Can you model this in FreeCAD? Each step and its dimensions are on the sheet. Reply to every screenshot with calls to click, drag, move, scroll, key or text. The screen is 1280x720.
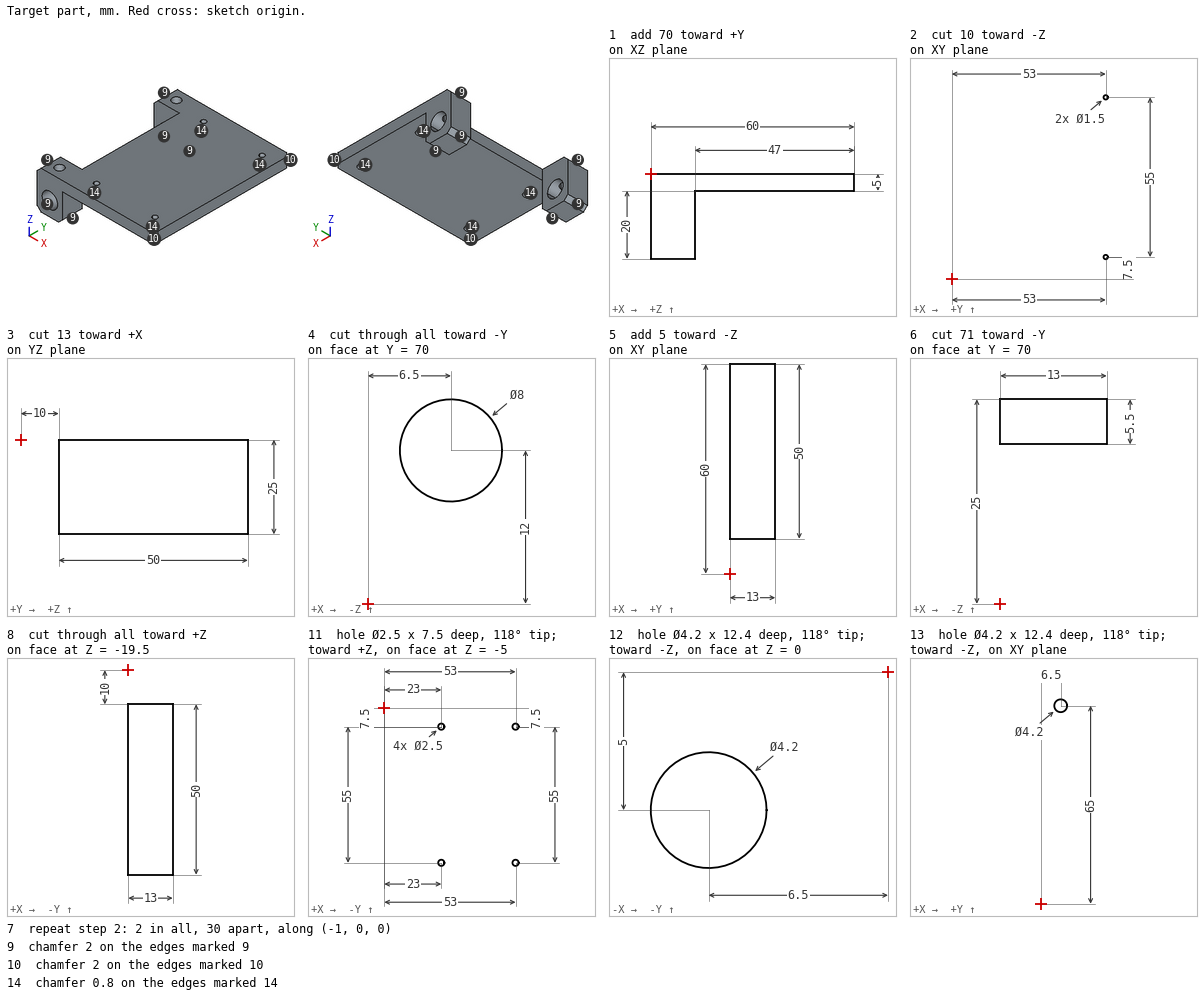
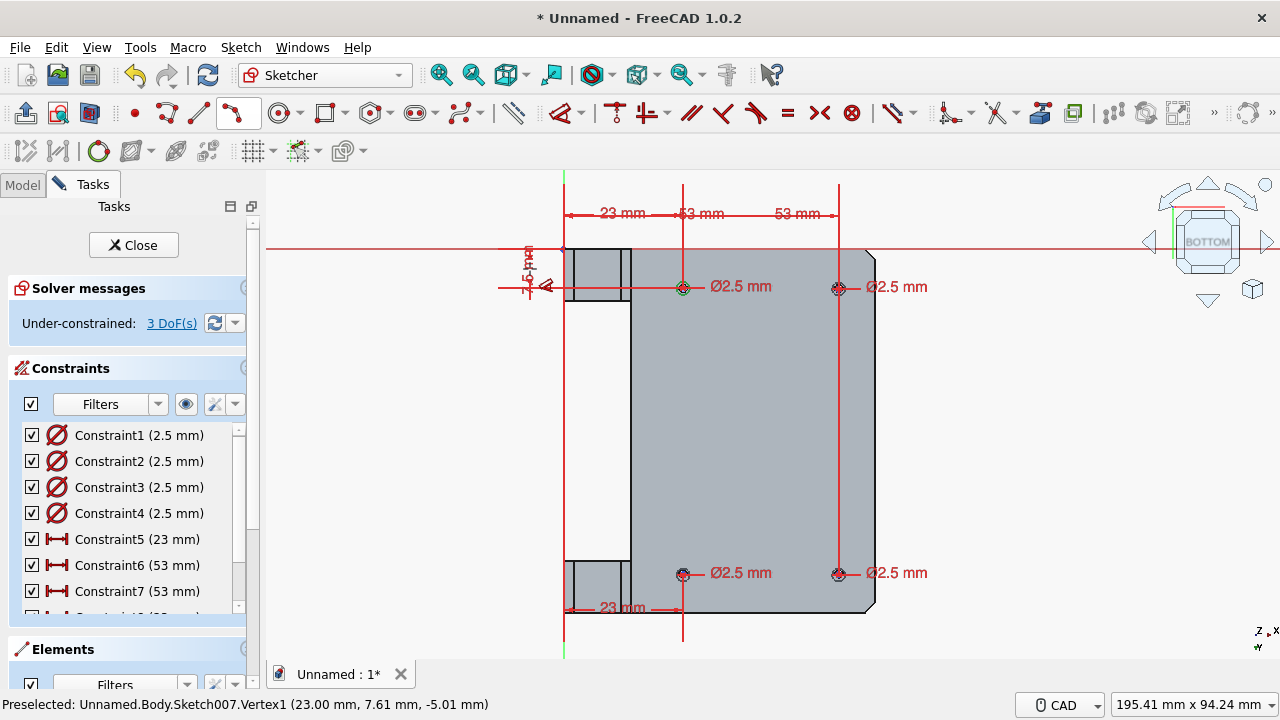
click(839, 289)
click(873, 269)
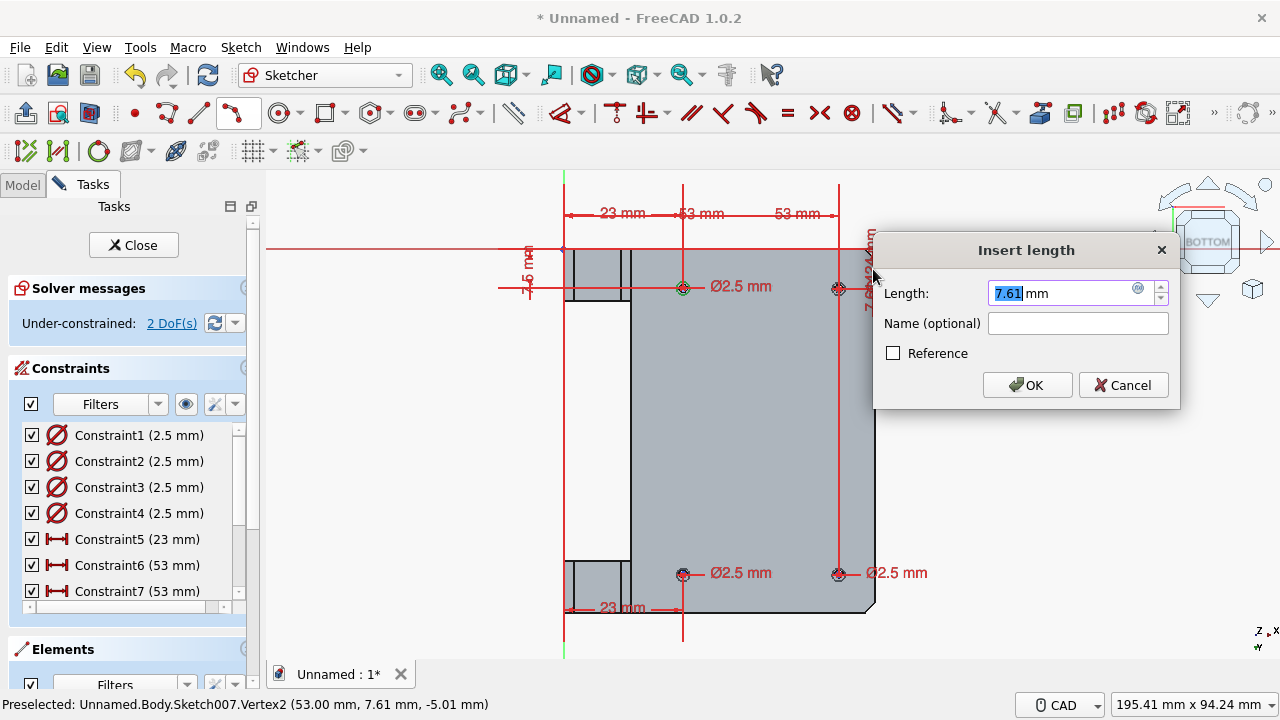
text(7.5)
key(Return)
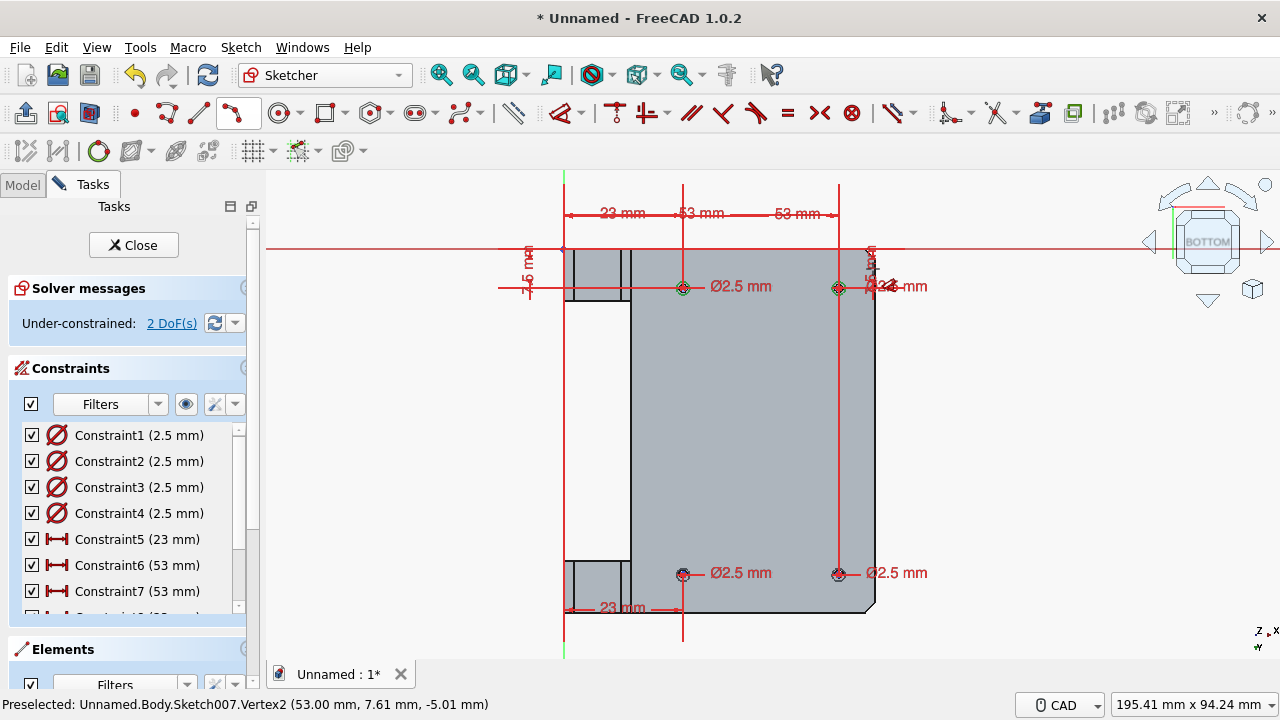
click(839, 288)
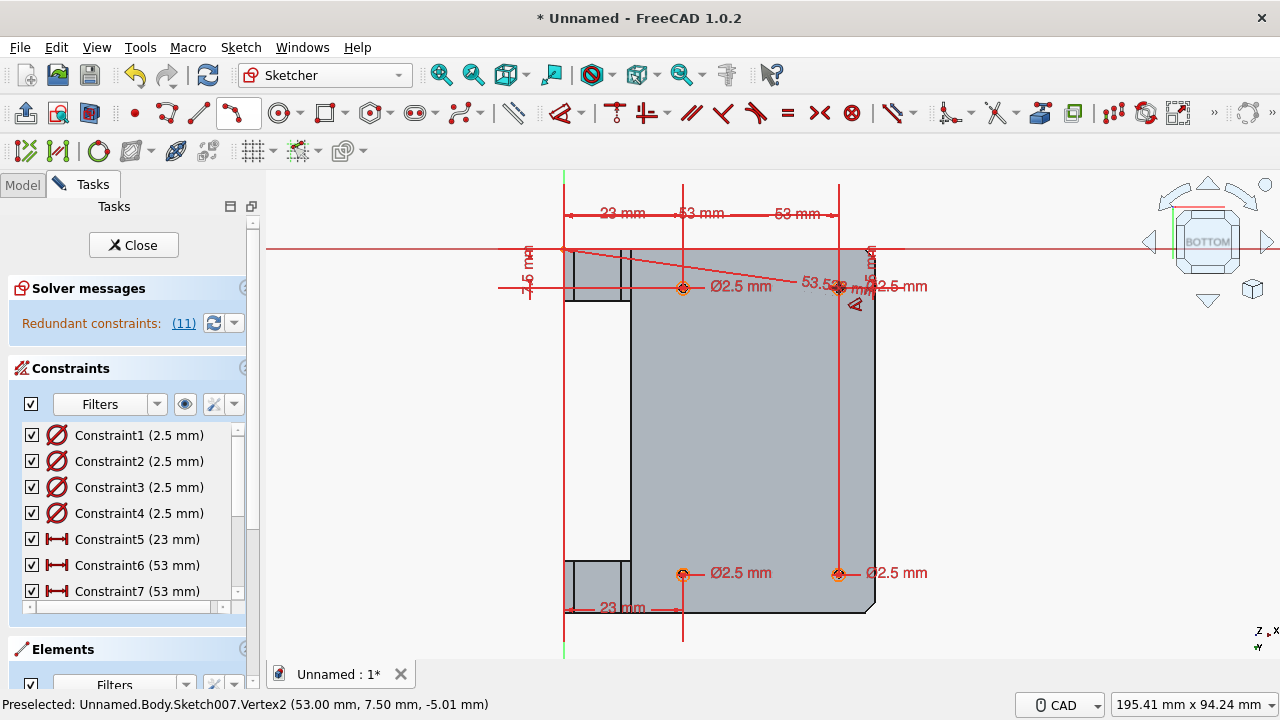
click(839, 575)
click(873, 432)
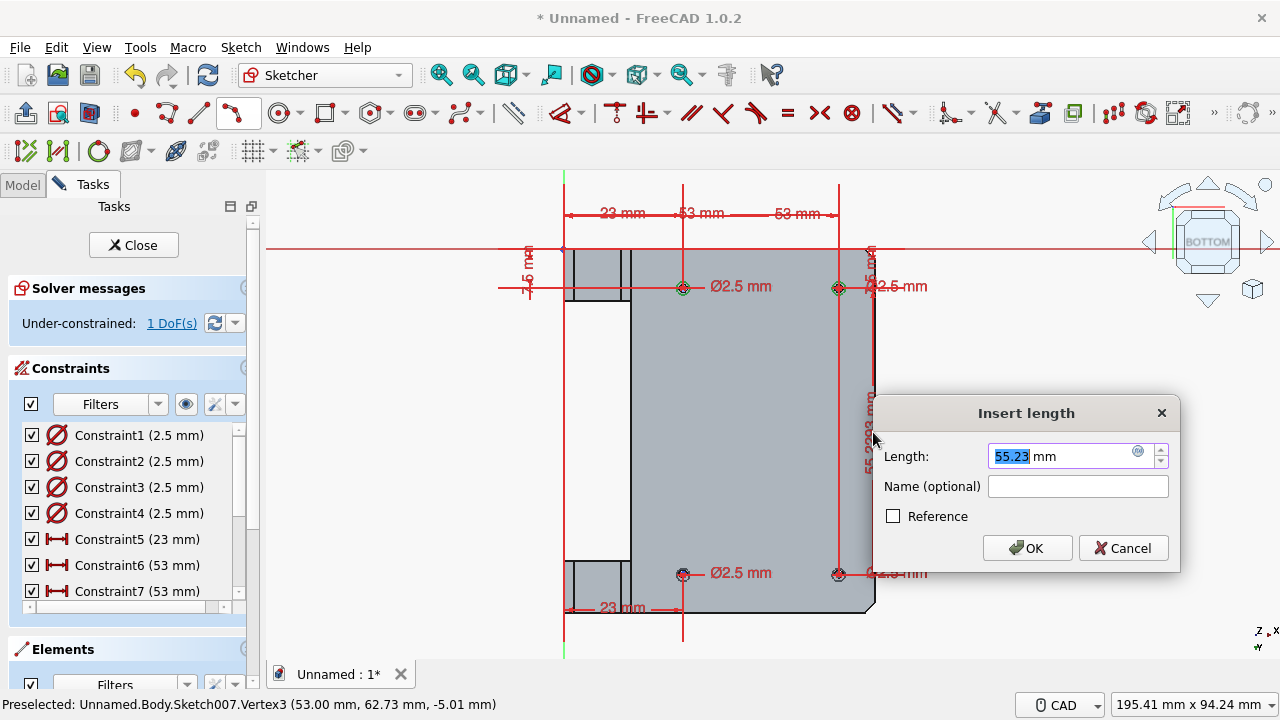
text(55)
key(Return)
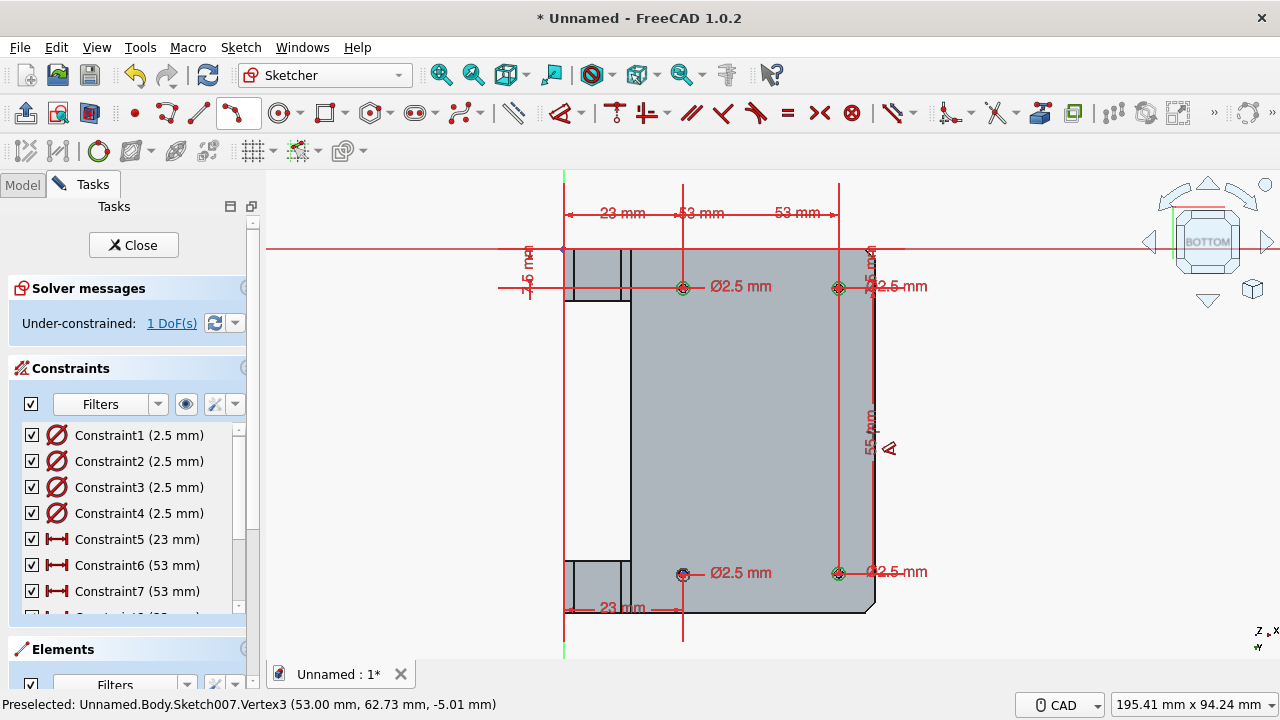
click(683, 288)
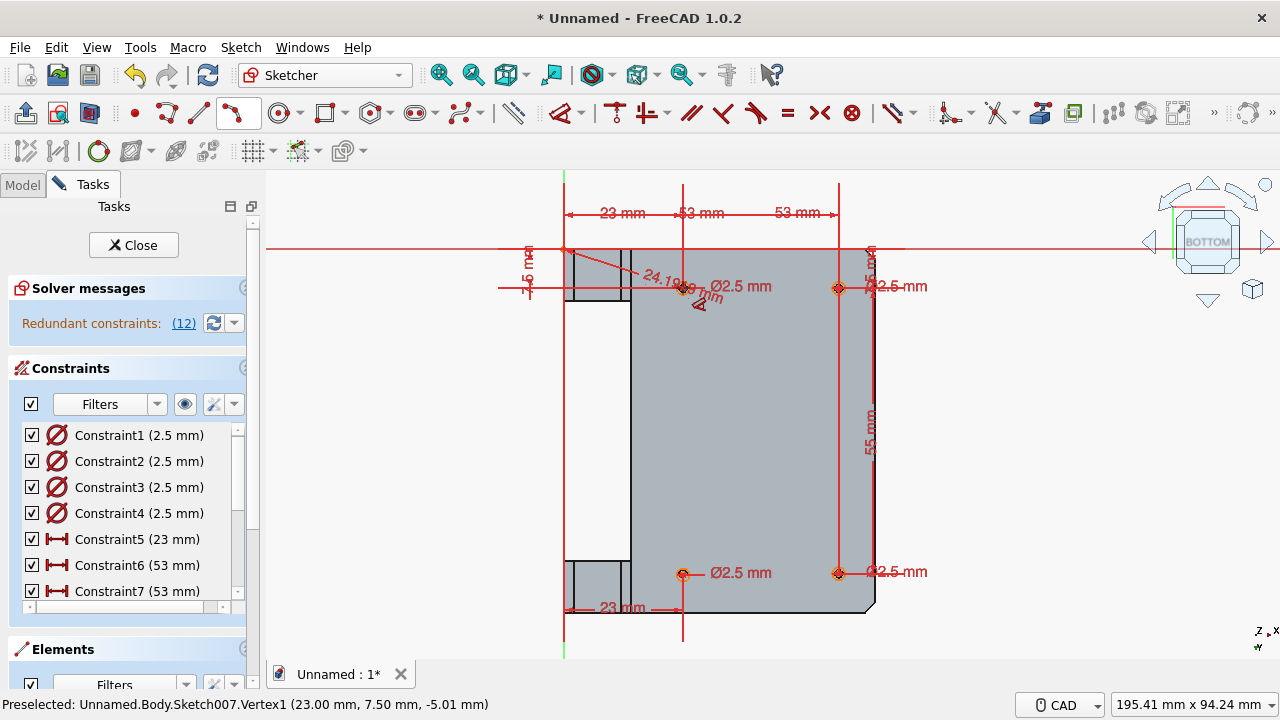
click(683, 575)
click(649, 432)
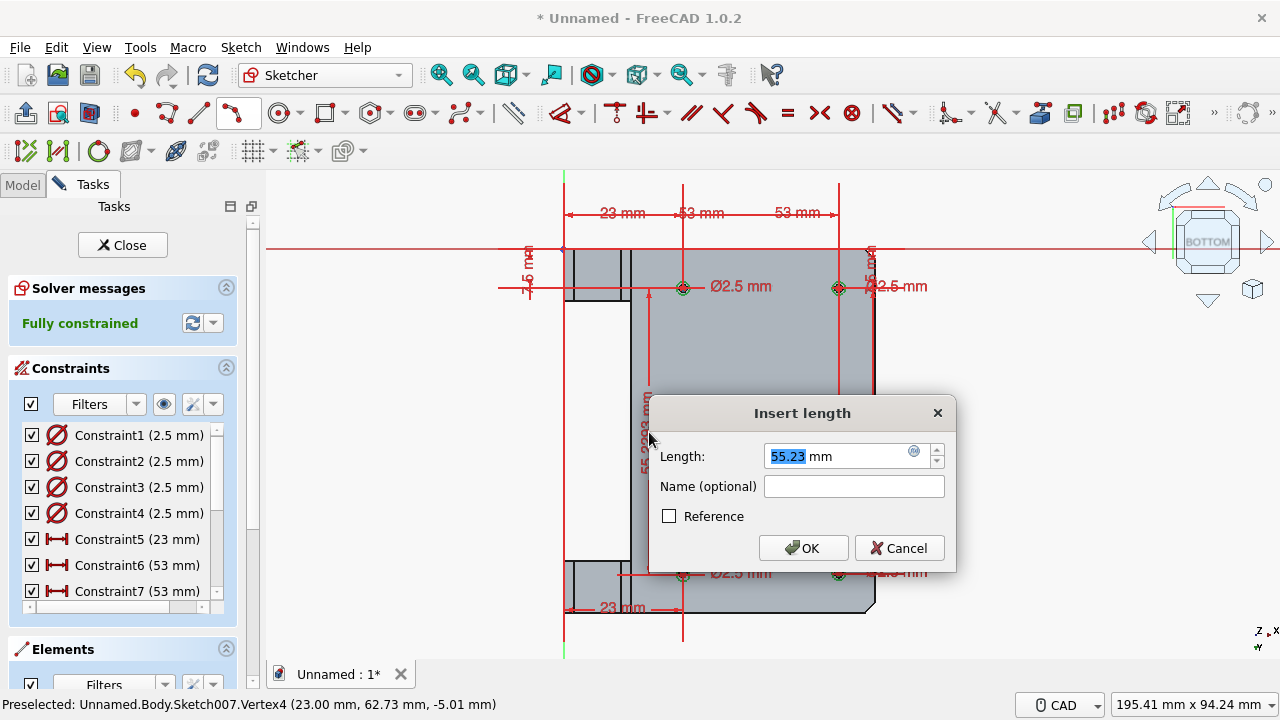
text(55)
key(Return)
key(Escape)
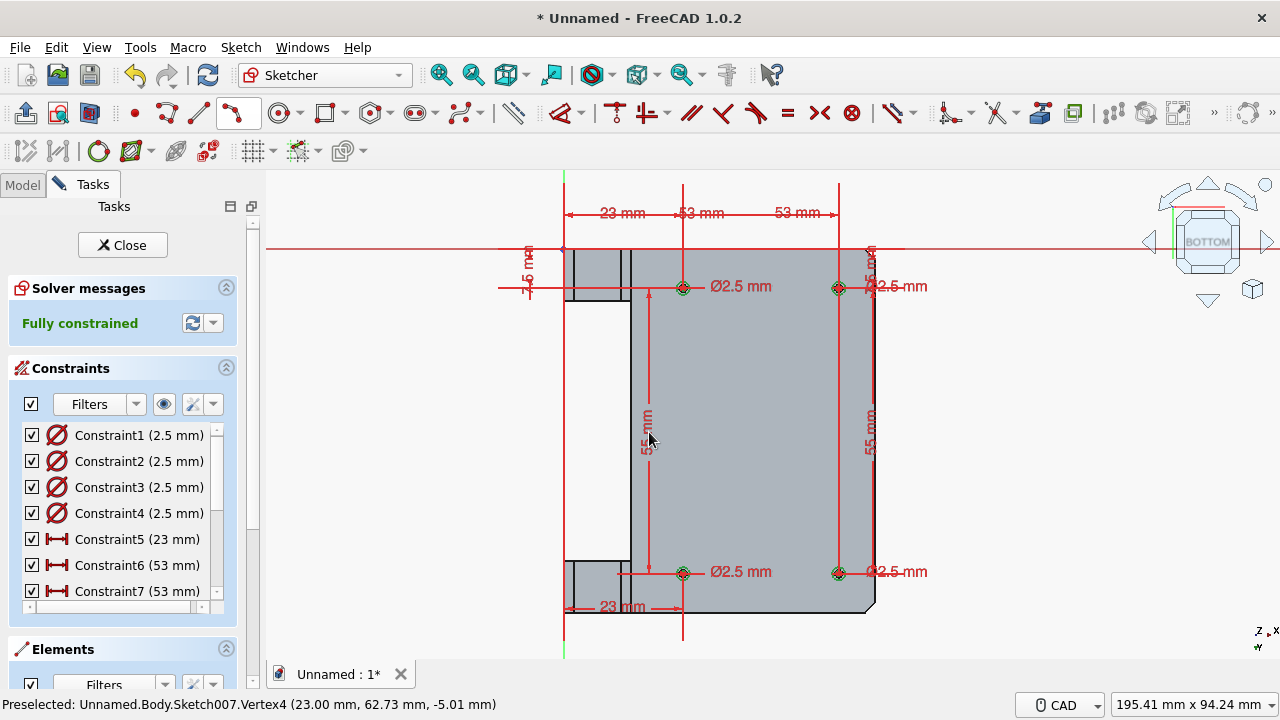
click(123, 245)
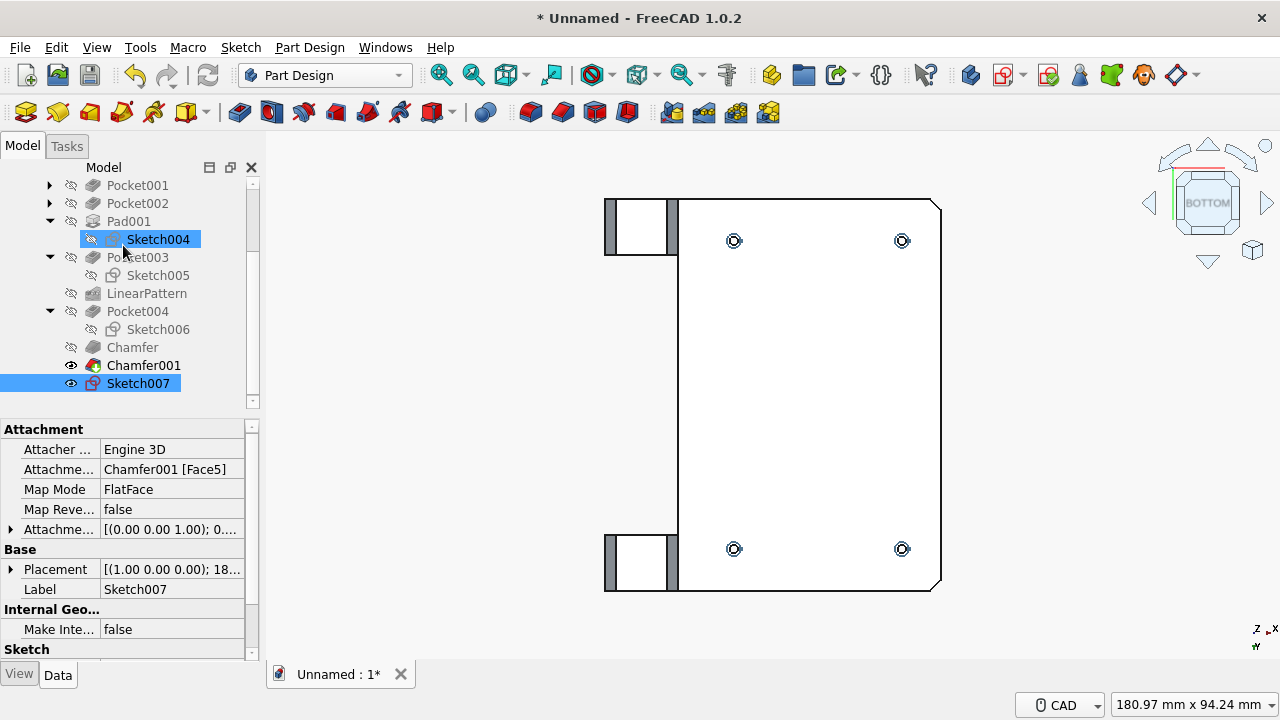
click(272, 112)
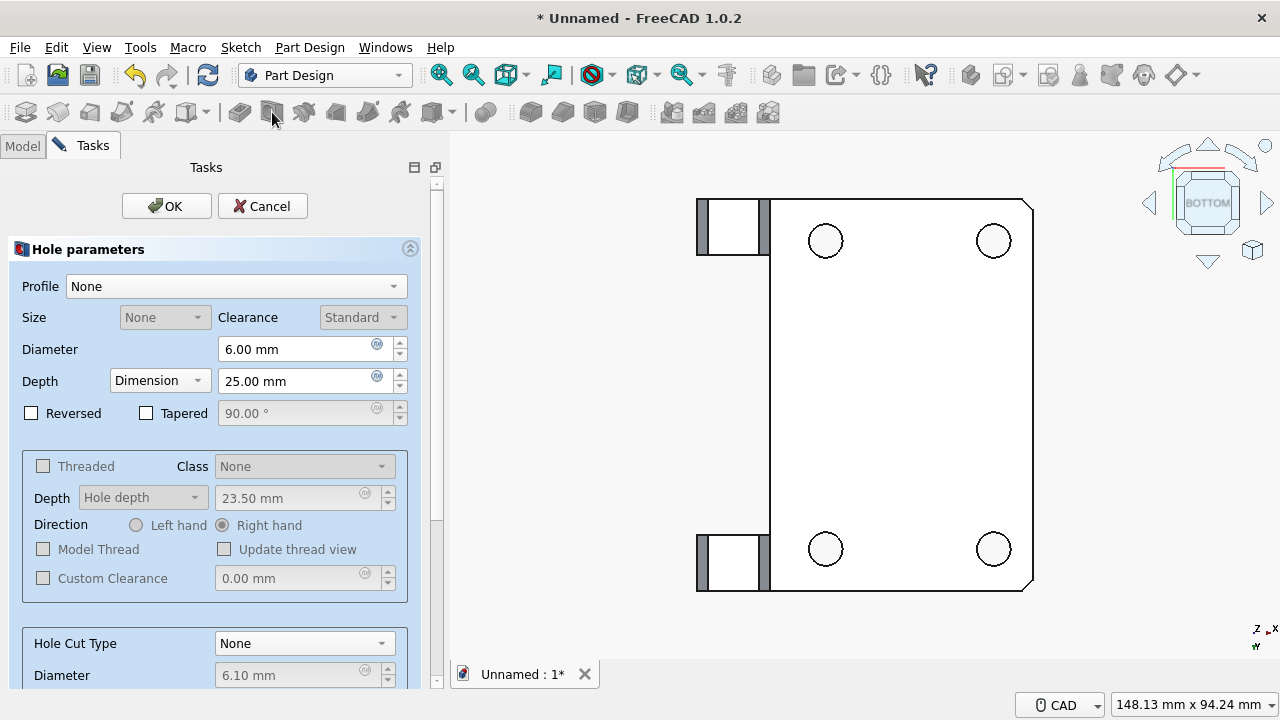
triple_click(305, 349)